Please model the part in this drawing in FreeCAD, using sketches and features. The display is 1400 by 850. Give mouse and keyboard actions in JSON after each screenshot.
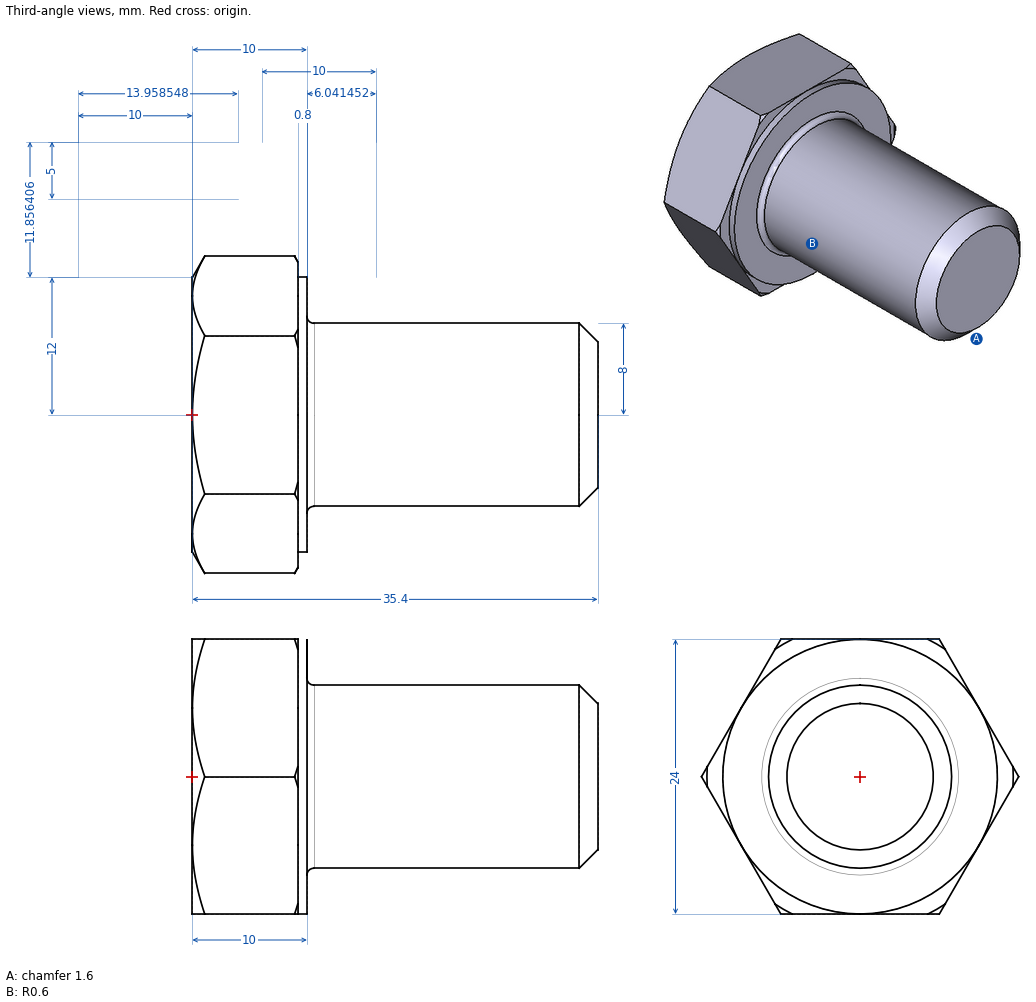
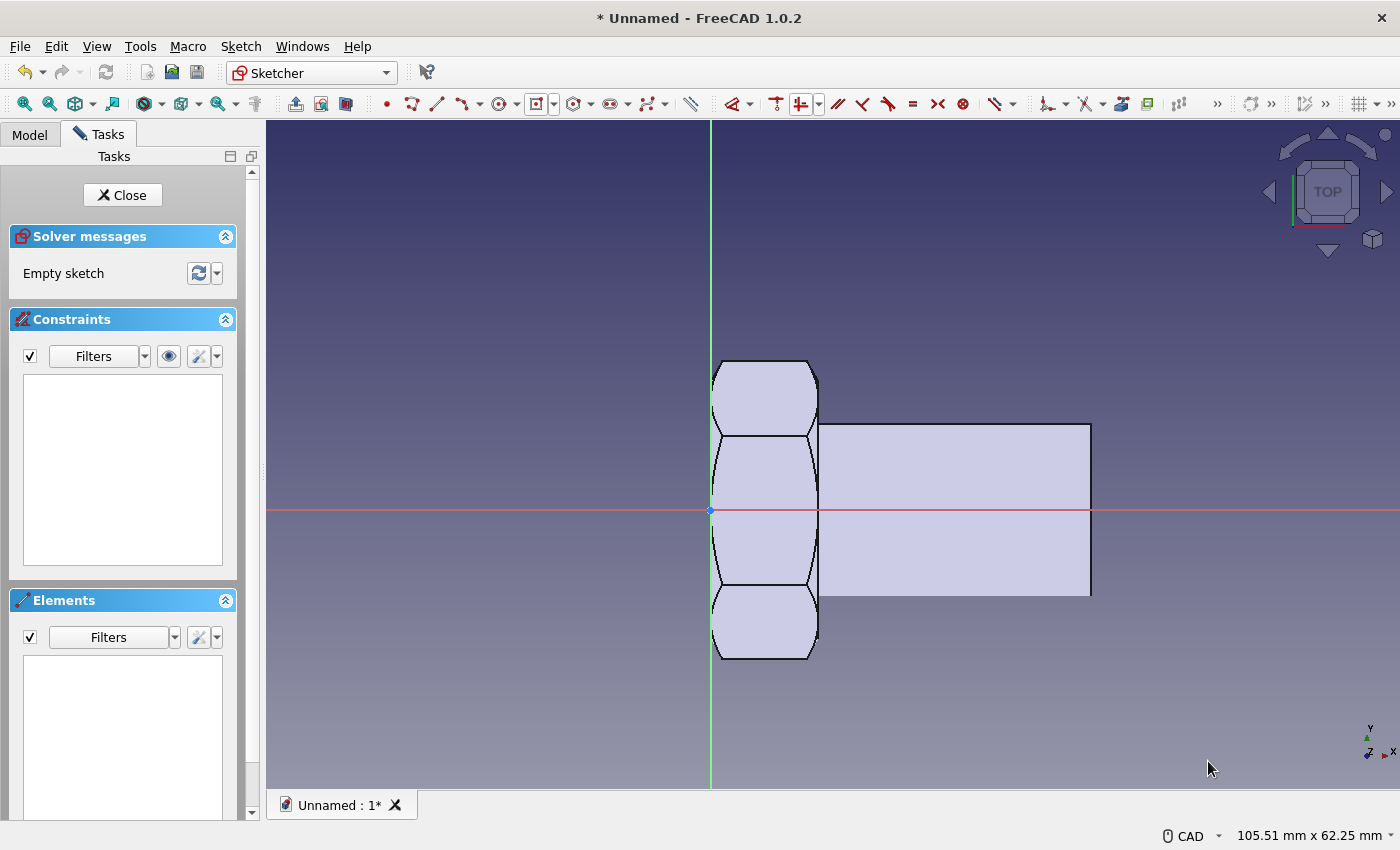
{"action": "scroll", "coordinate": [765, 294], "scroll_direction": "up", "scroll_amount": 3}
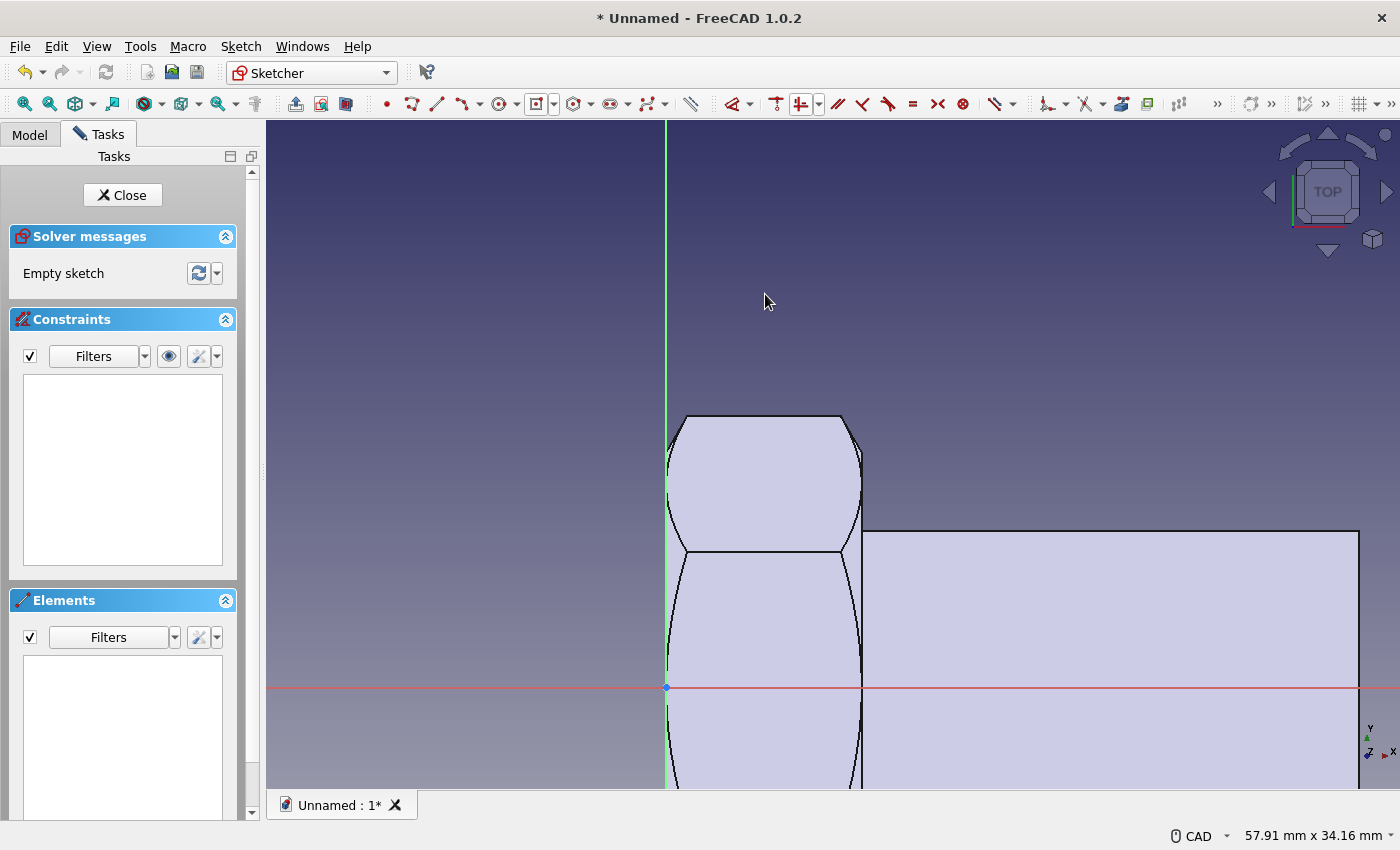
{"action": "key", "text": "g r"}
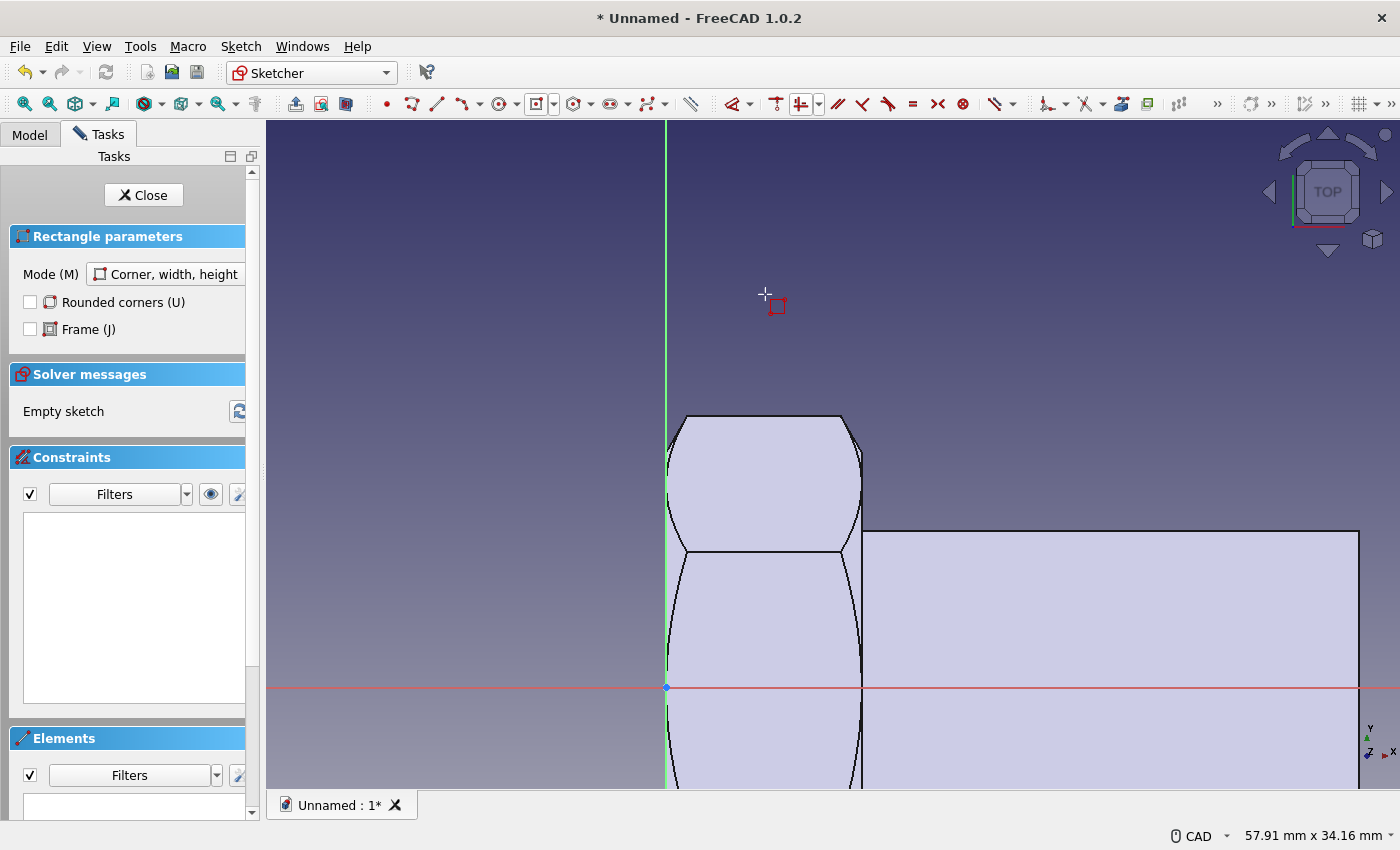
{"action": "left_click", "coordinate": [846, 221]}
{"action": "mouse_move", "coordinate": [862, 453]}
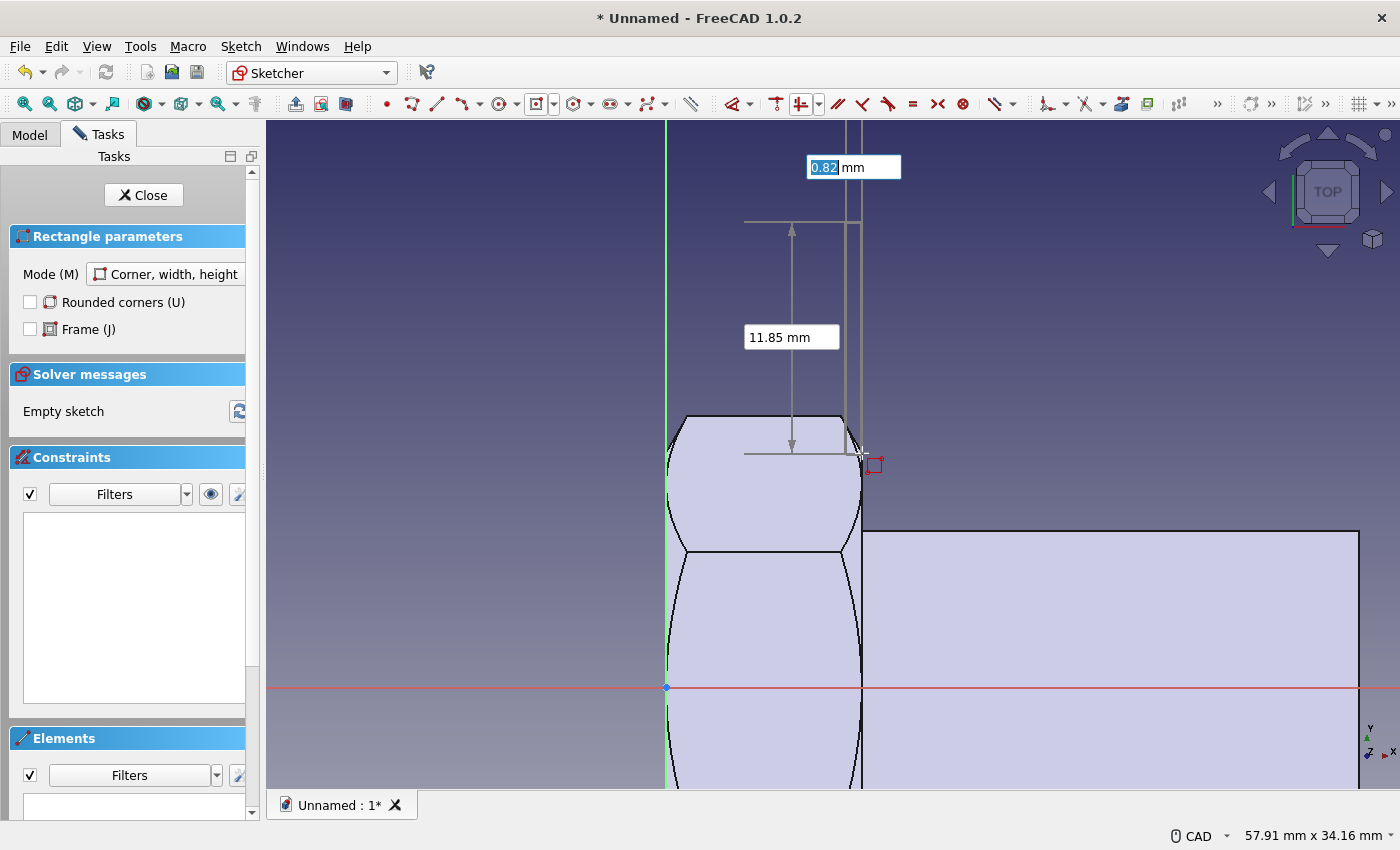
{"action": "type", "text": "0.8"}
{"action": "key", "text": "Tab"}
{"action": "type", "text": "11.856406"}
{"action": "key", "text": "Return"}
{"action": "key", "text": "Escape"}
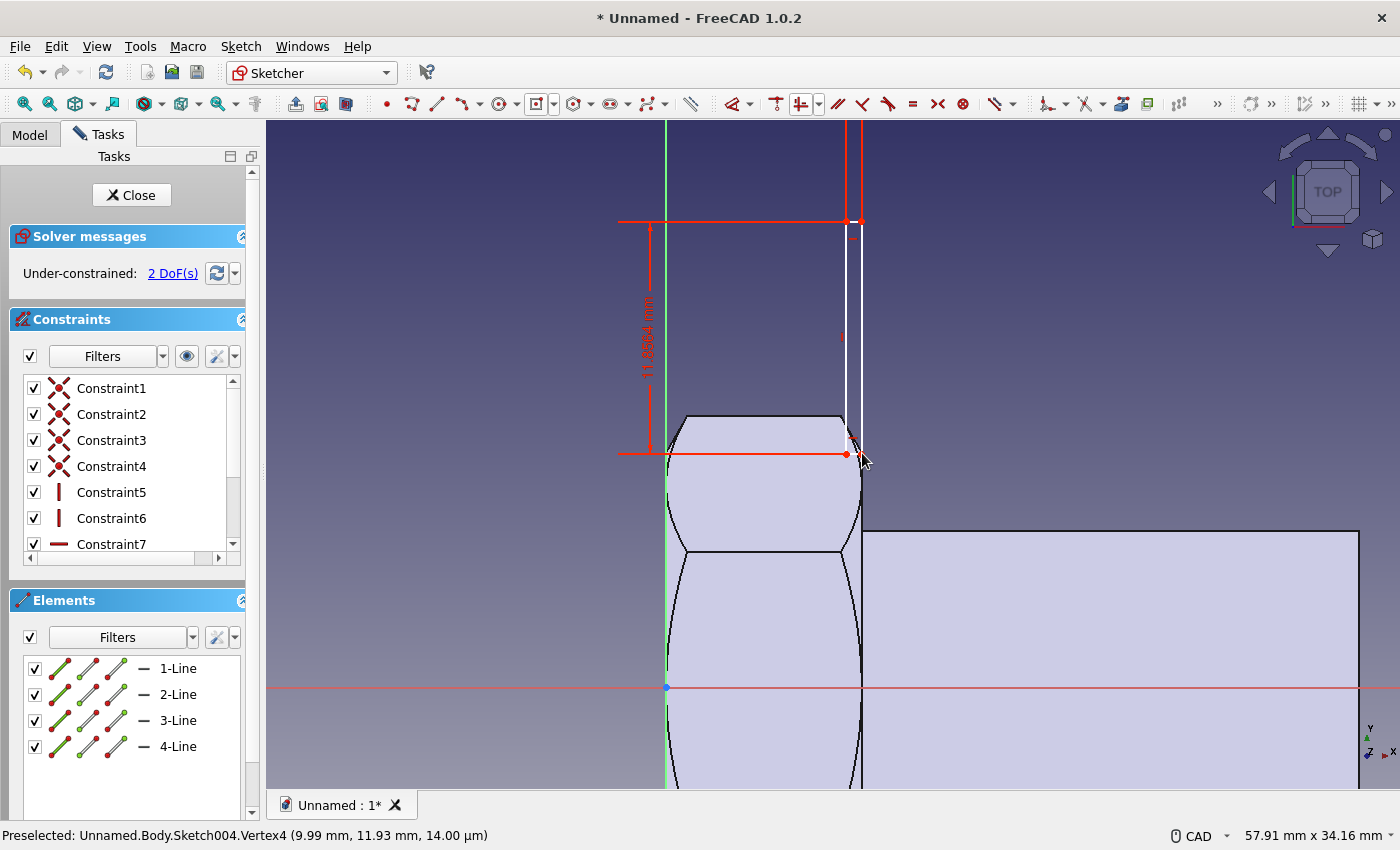
{"action": "left_click", "coordinate": [732, 104]}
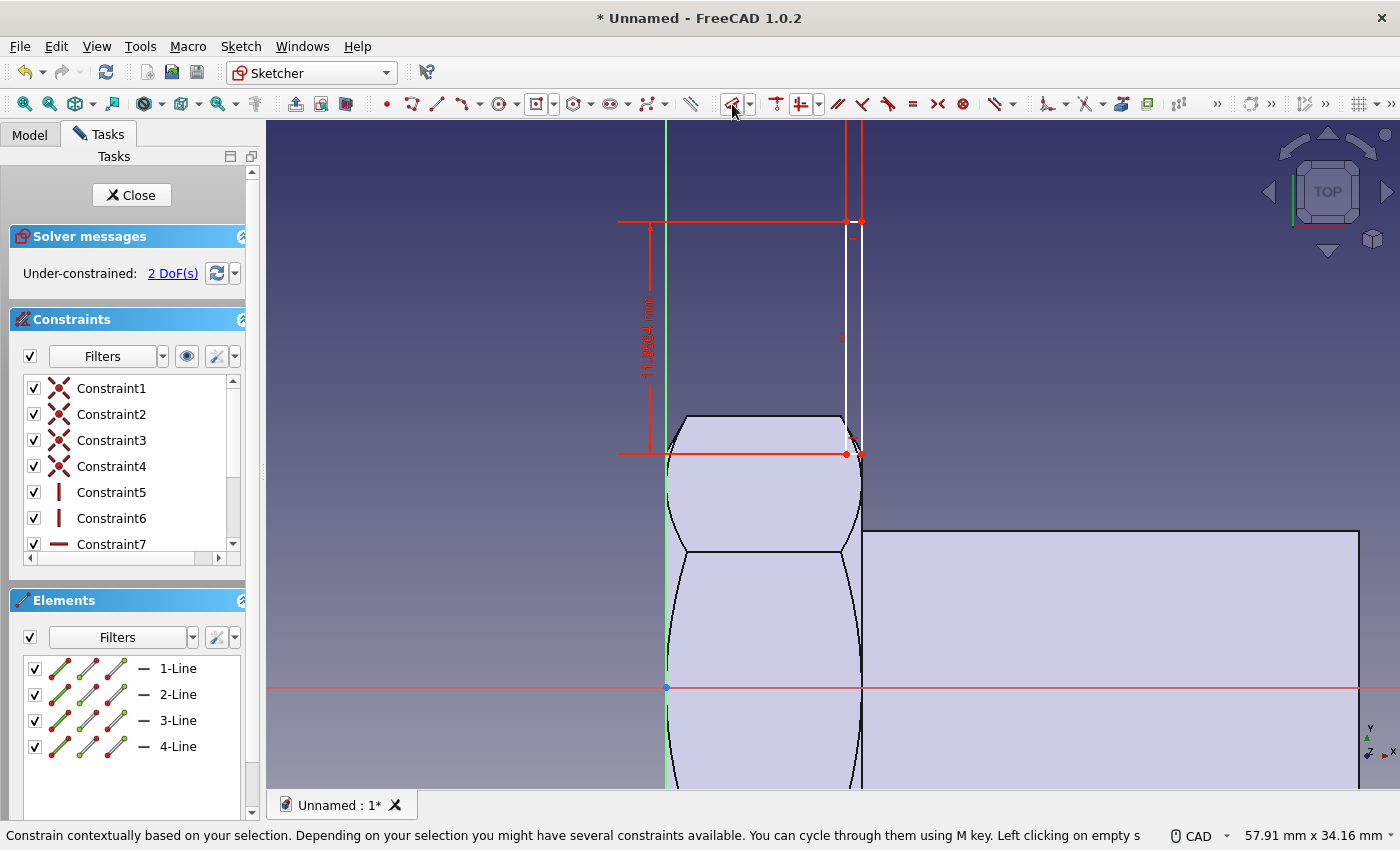
{"action": "left_click", "coordinate": [846, 454]}
{"action": "left_click", "coordinate": [632, 571]}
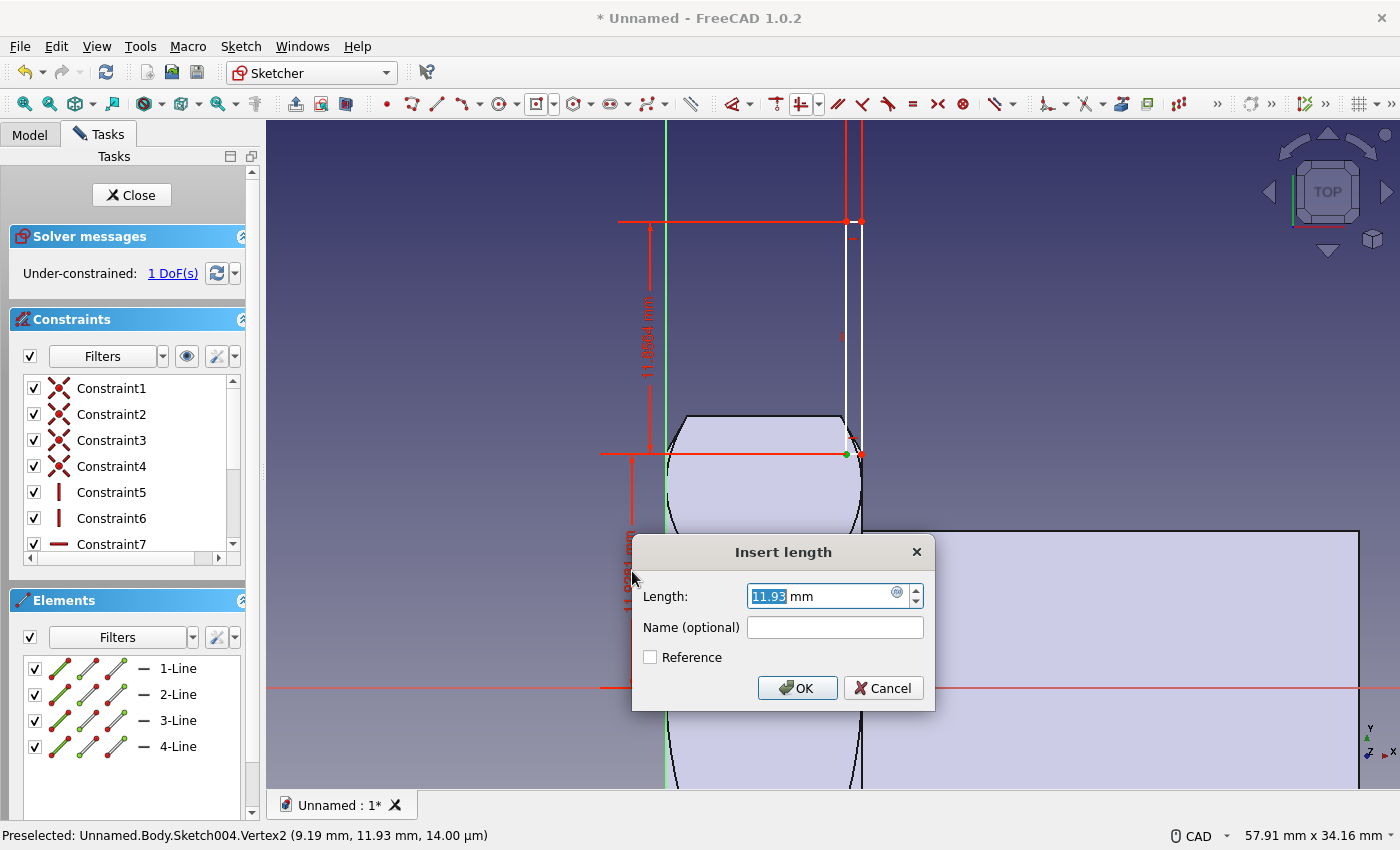
{"action": "type", "text": "12"}
{"action": "key", "text": "Return"}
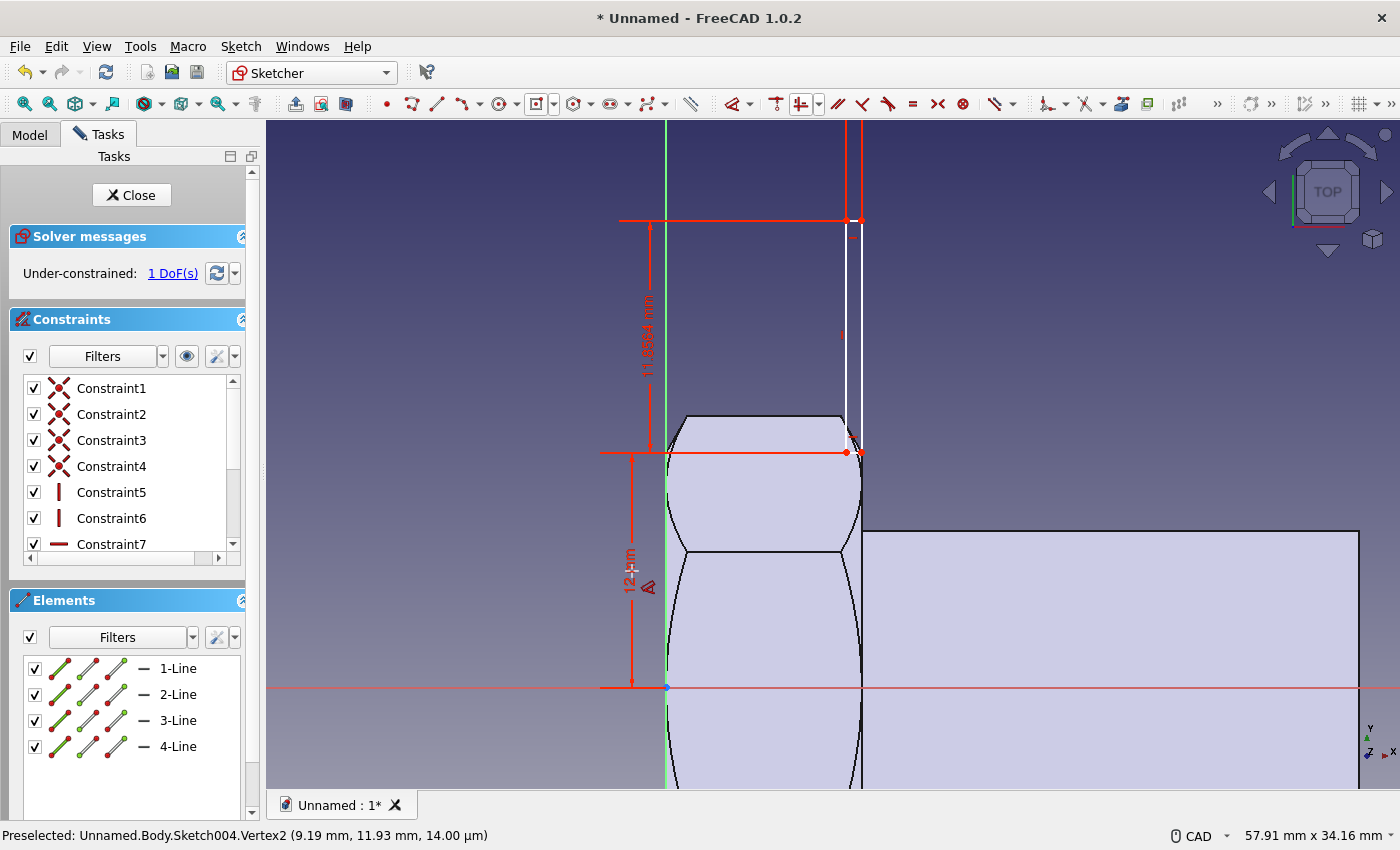
{"action": "left_click", "coordinate": [862, 453]}
{"action": "left_click", "coordinate": [764, 722]}